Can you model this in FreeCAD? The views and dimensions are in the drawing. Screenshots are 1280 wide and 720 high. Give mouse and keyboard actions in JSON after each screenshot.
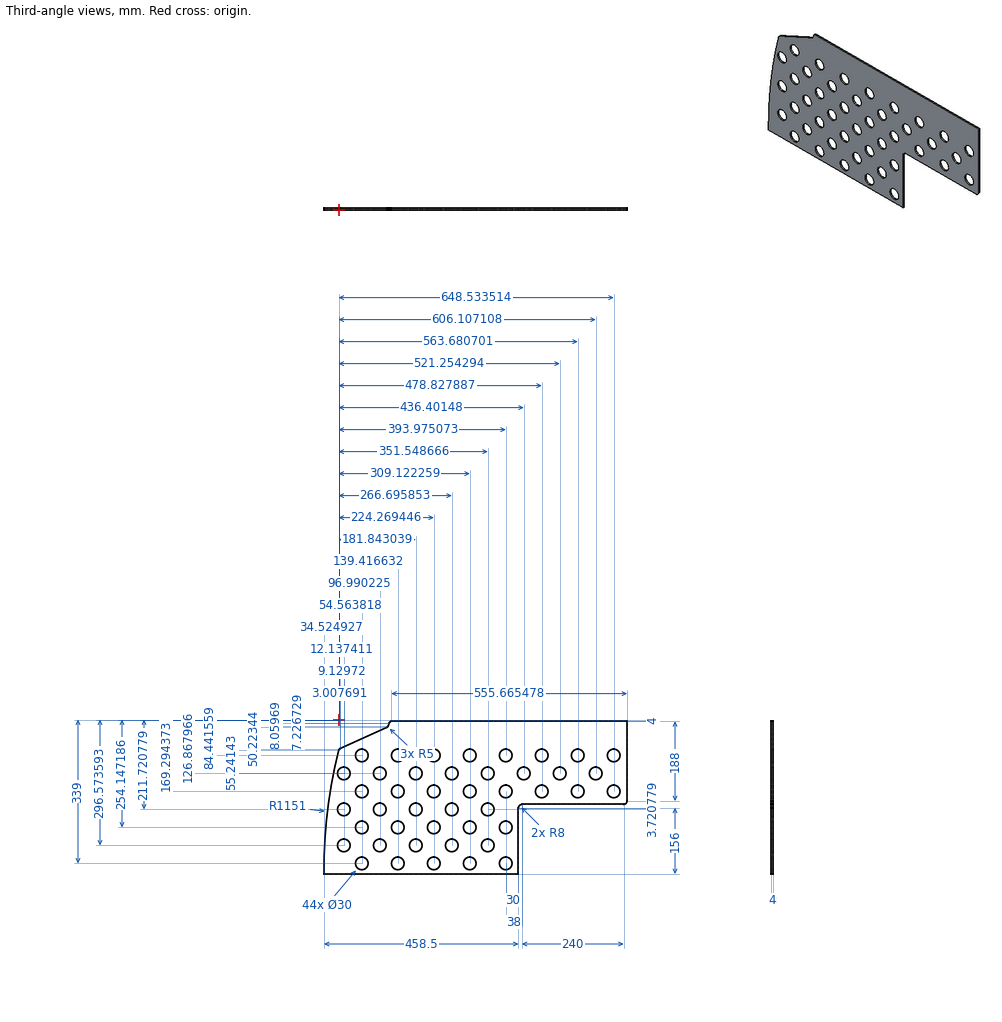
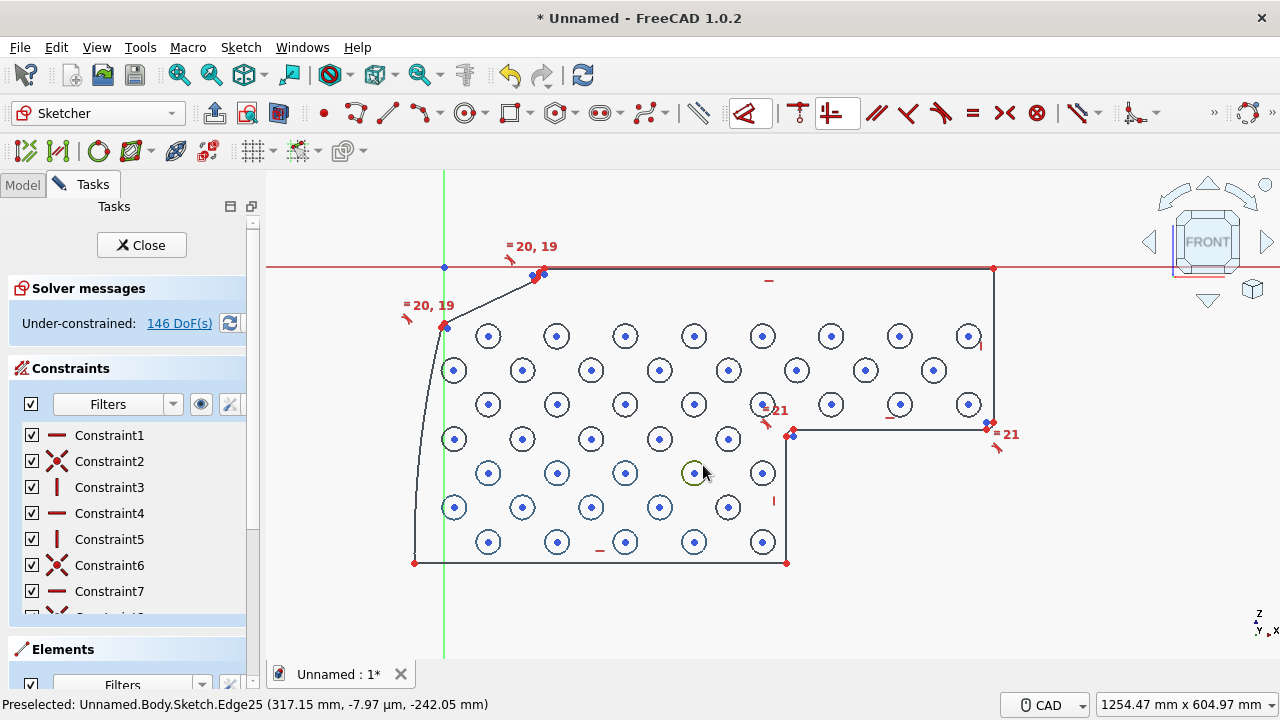
{"action": "left_click", "coordinate": [771, 534]}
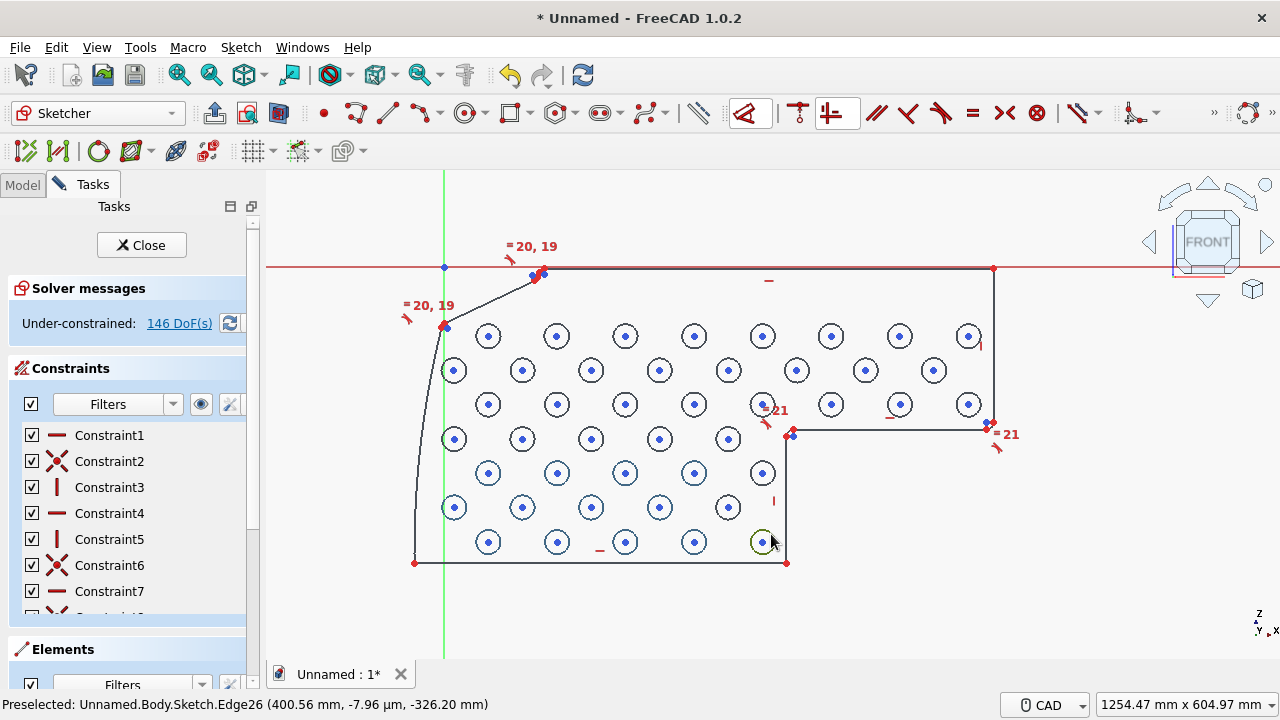
{"action": "left_click", "coordinate": [737, 499]}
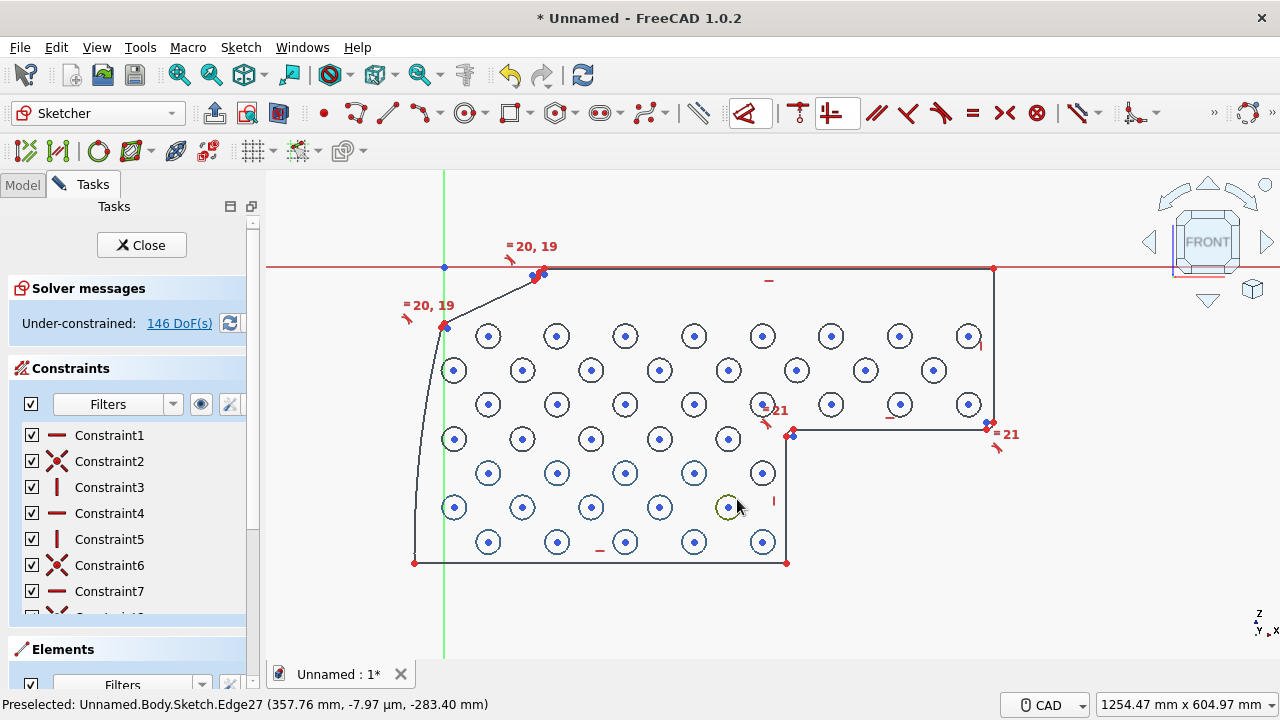
{"action": "left_click", "coordinate": [771, 465]}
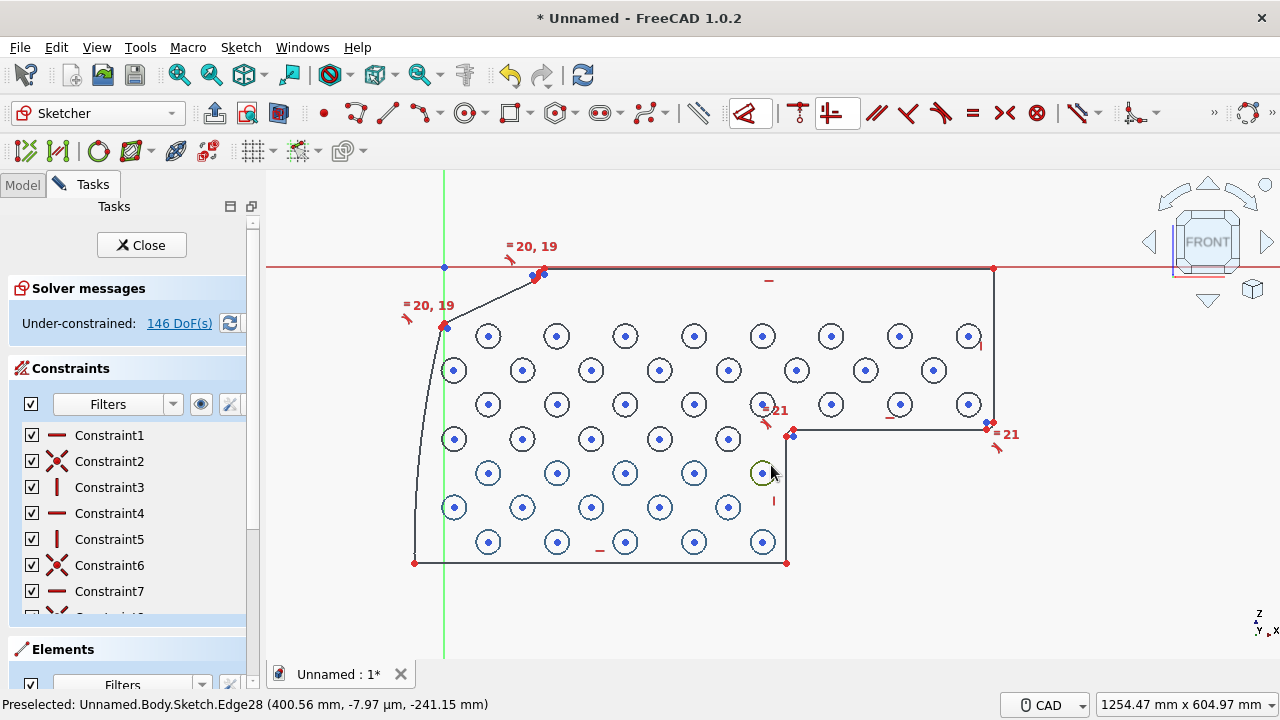
{"action": "left_click", "coordinate": [463, 431]}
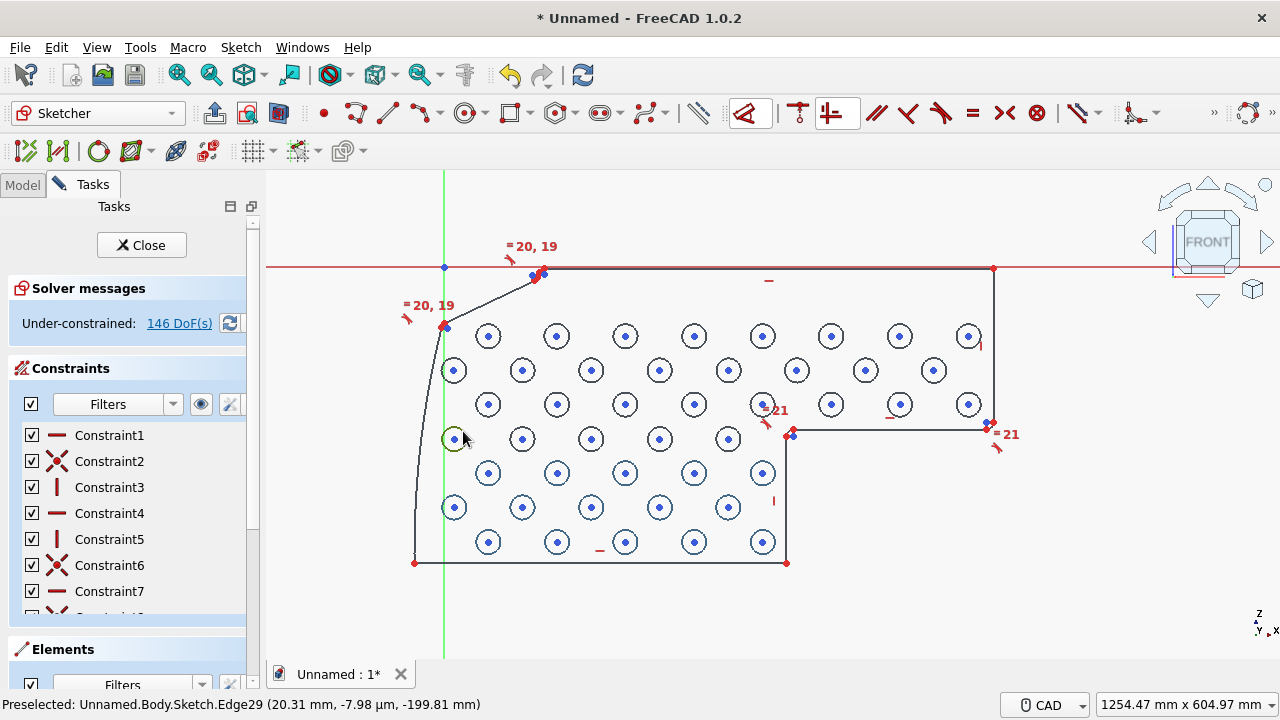
{"action": "left_click", "coordinate": [531, 431]}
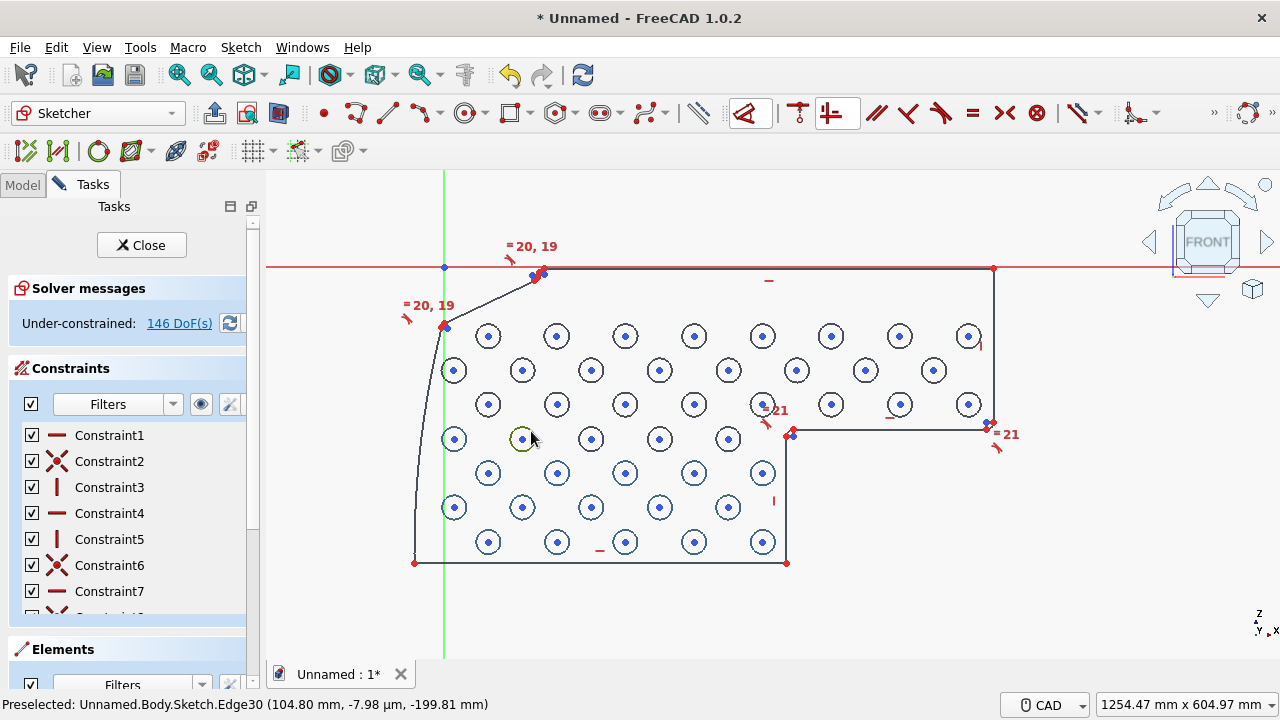
{"action": "left_click", "coordinate": [497, 396]}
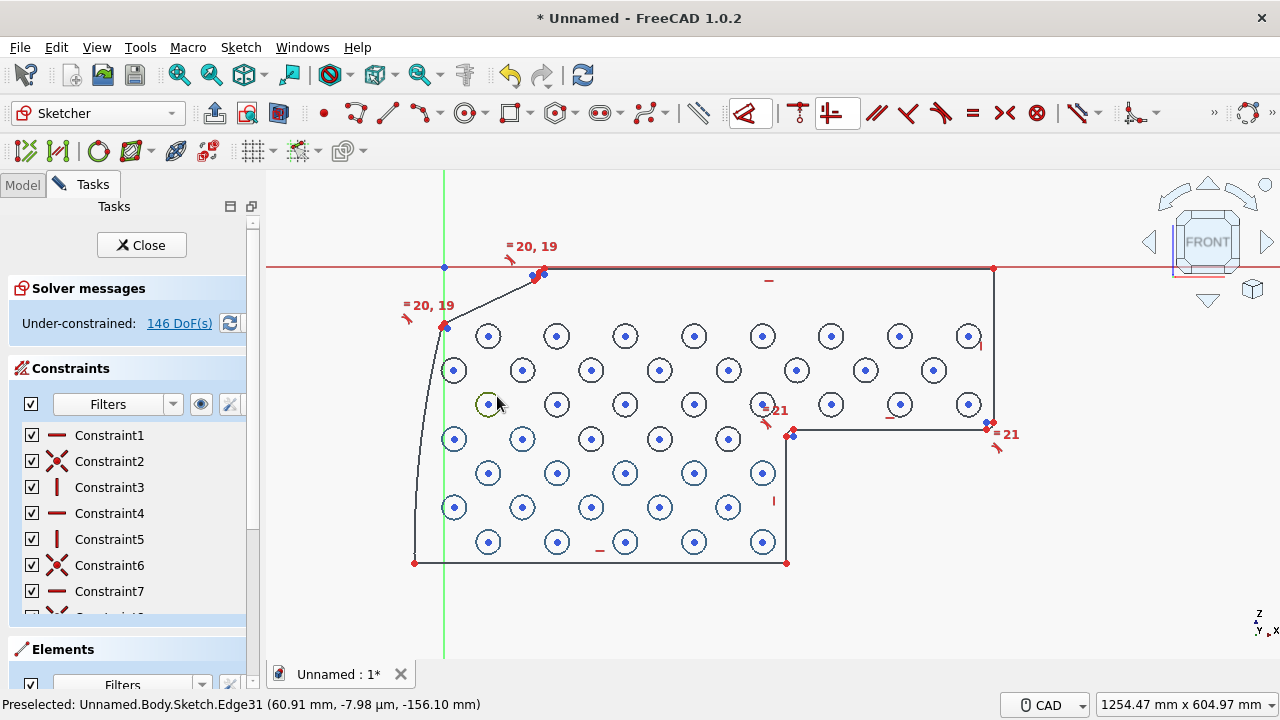
{"action": "left_click", "coordinate": [566, 396]}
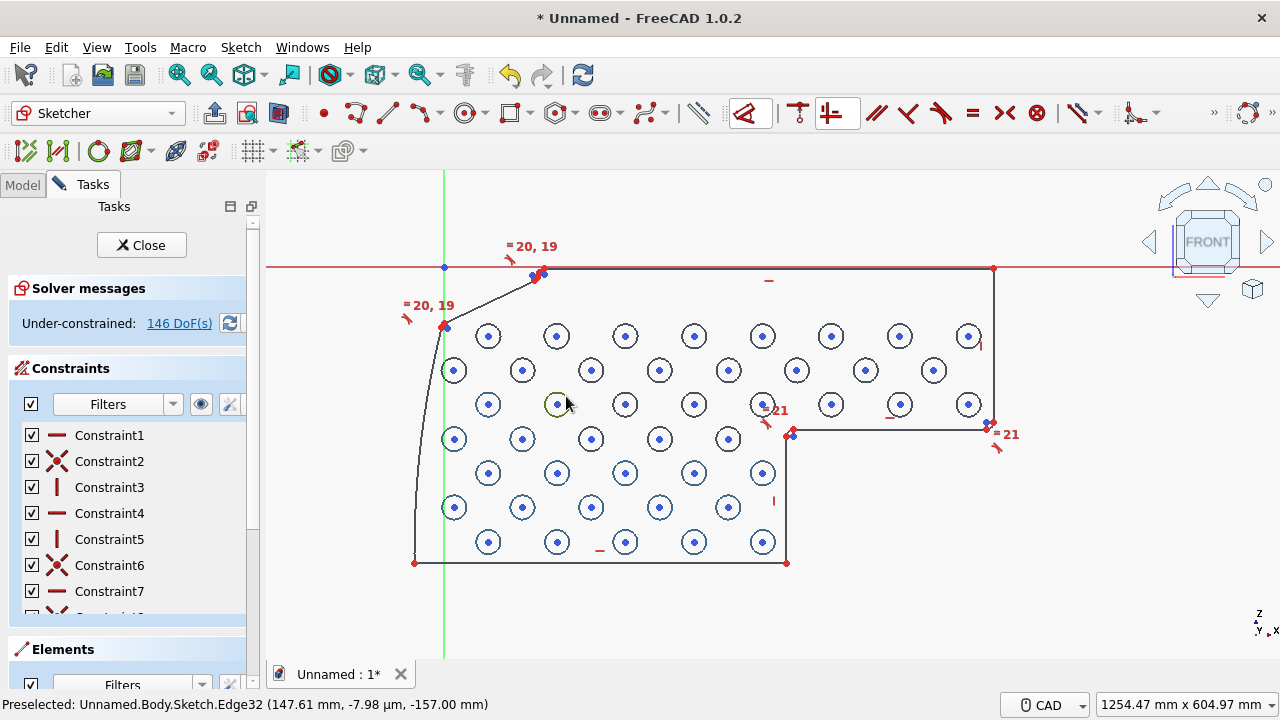
{"action": "left_click", "coordinate": [600, 431]}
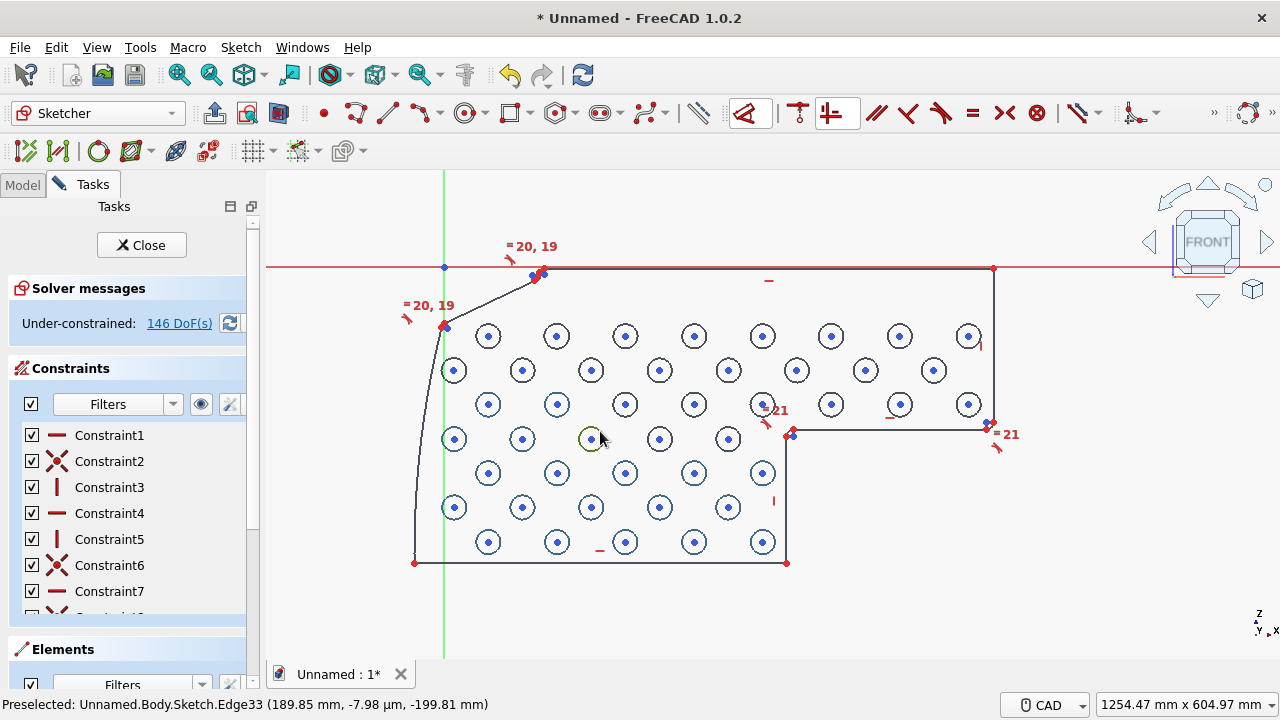
{"action": "left_click", "coordinate": [669, 431]}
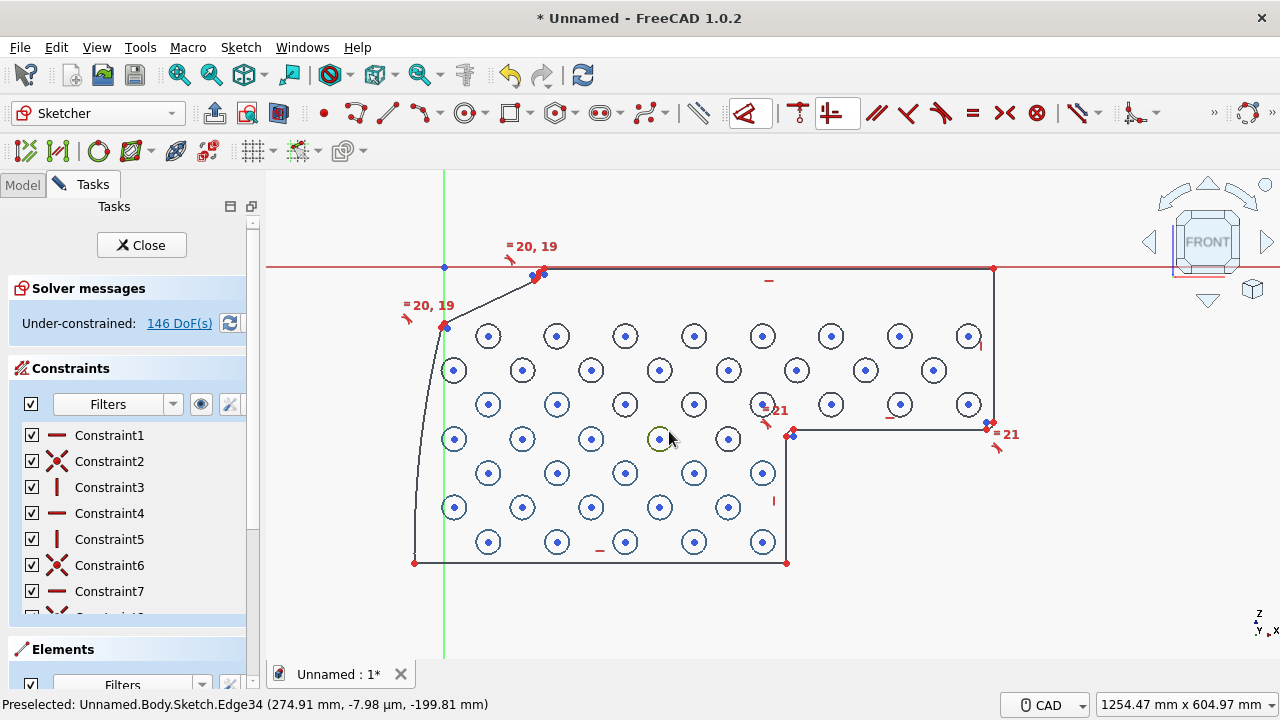
{"action": "left_click", "coordinate": [634, 396]}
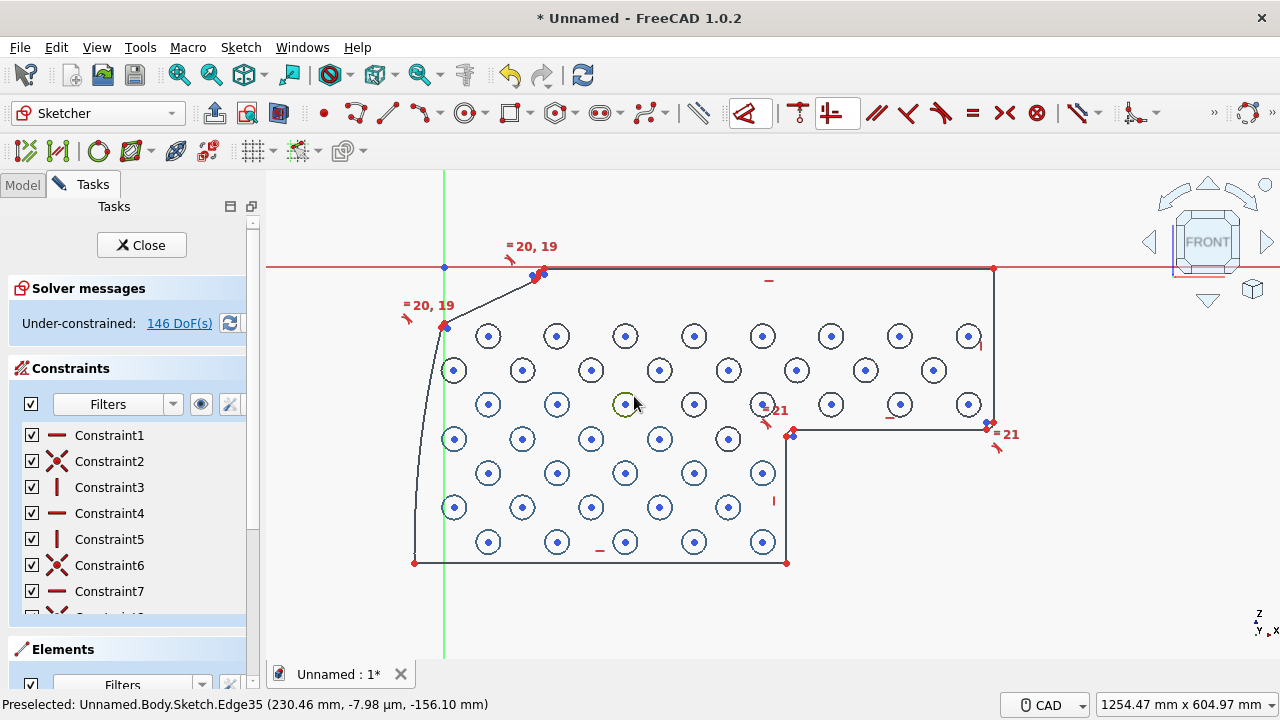
{"action": "left_click", "coordinate": [703, 396]}